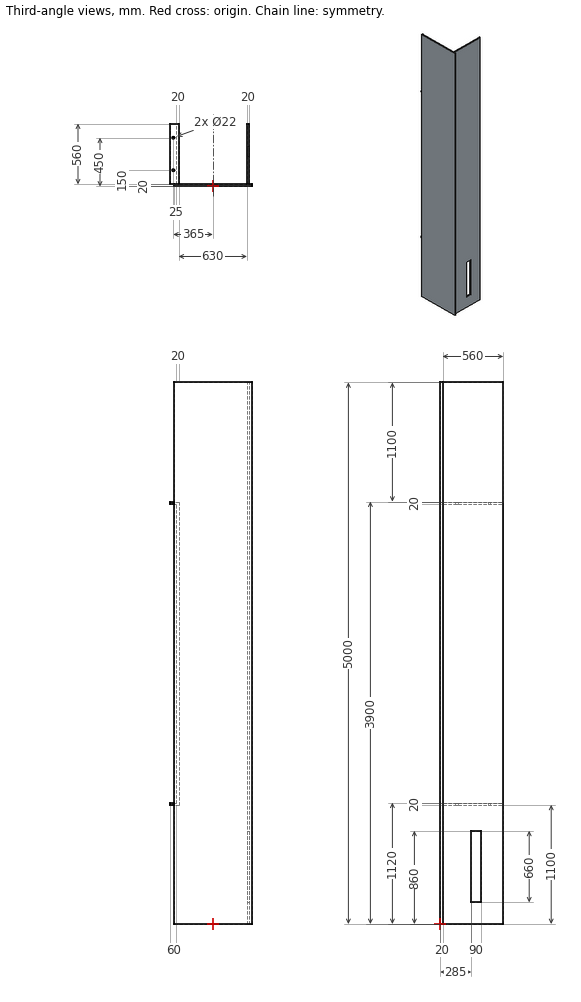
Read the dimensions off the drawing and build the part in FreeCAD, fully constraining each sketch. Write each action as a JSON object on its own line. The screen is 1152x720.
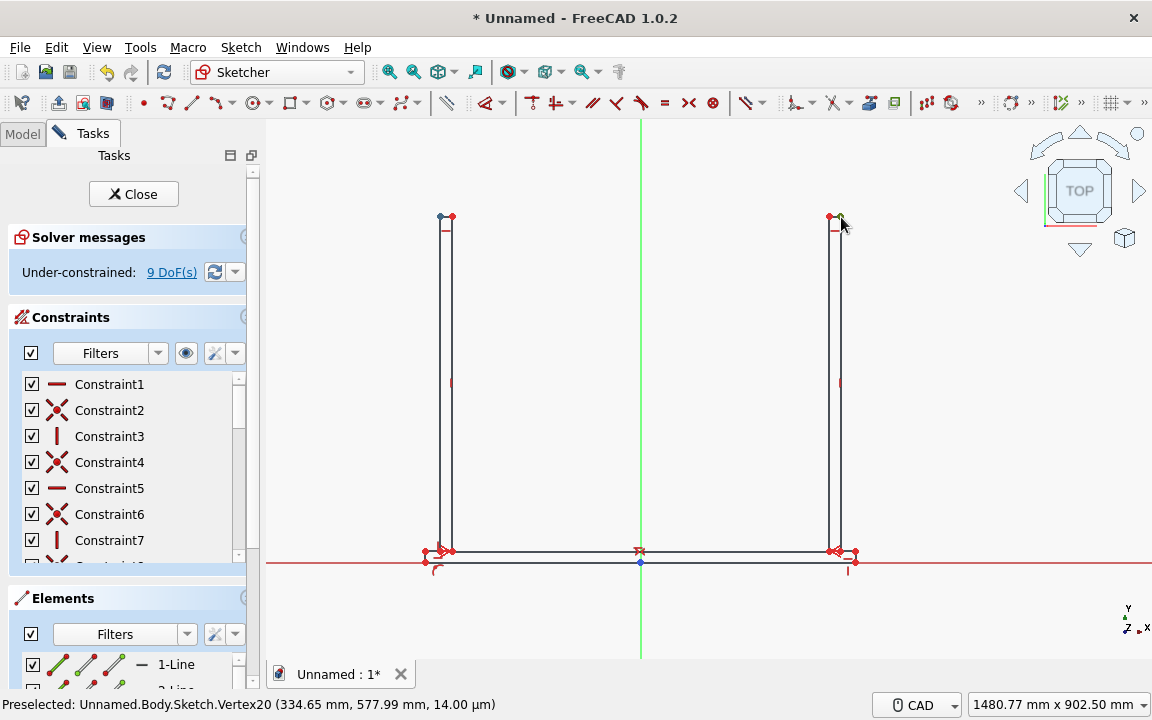
{"action": "left_click", "coordinate": [641, 596]}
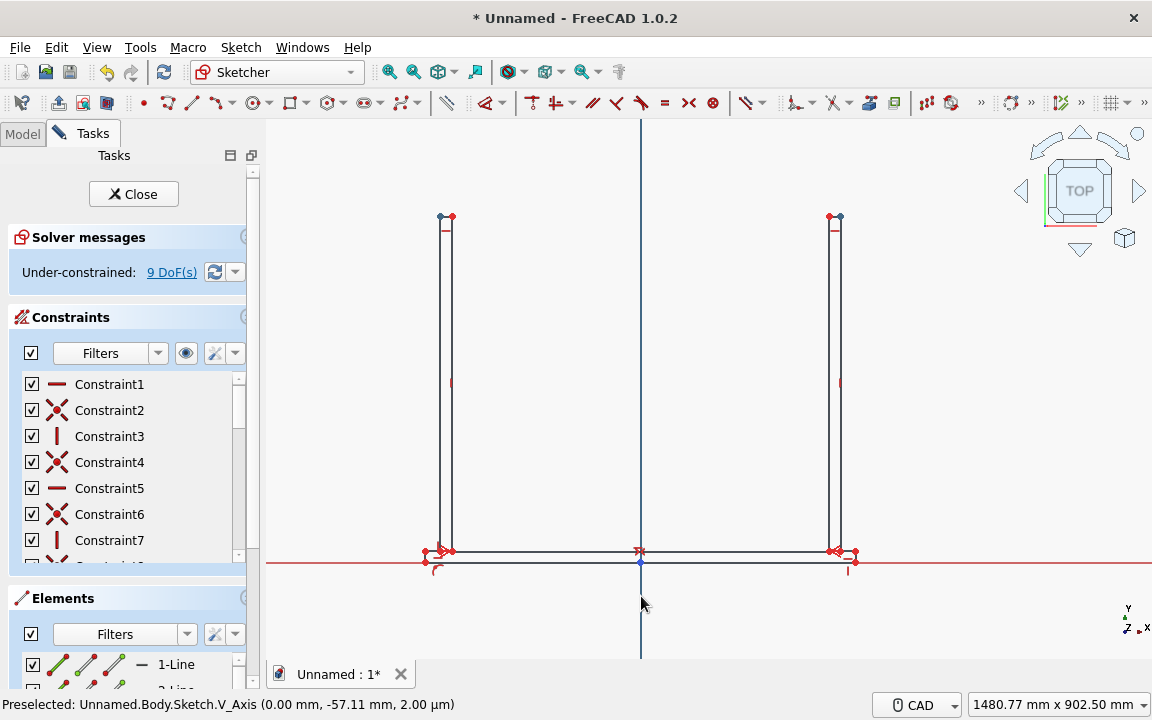
{"action": "left_click", "coordinate": [690, 104]}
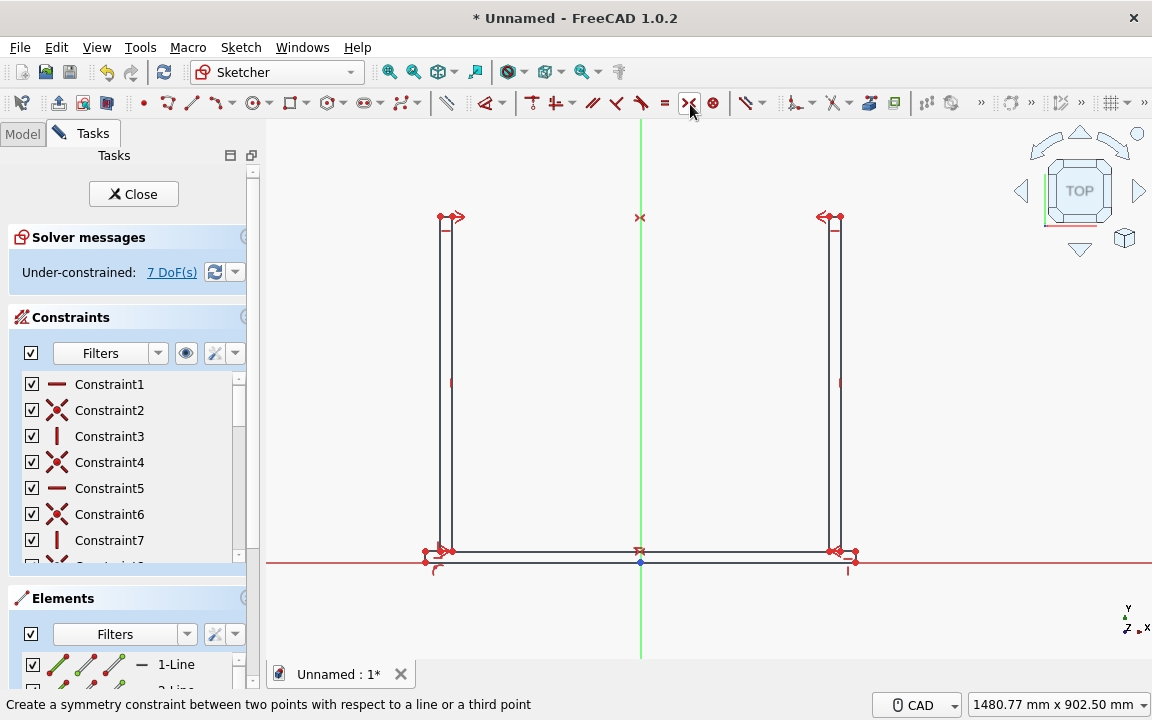
{"action": "scroll", "coordinate": [446, 217], "scroll_direction": "up", "scroll_amount": 6}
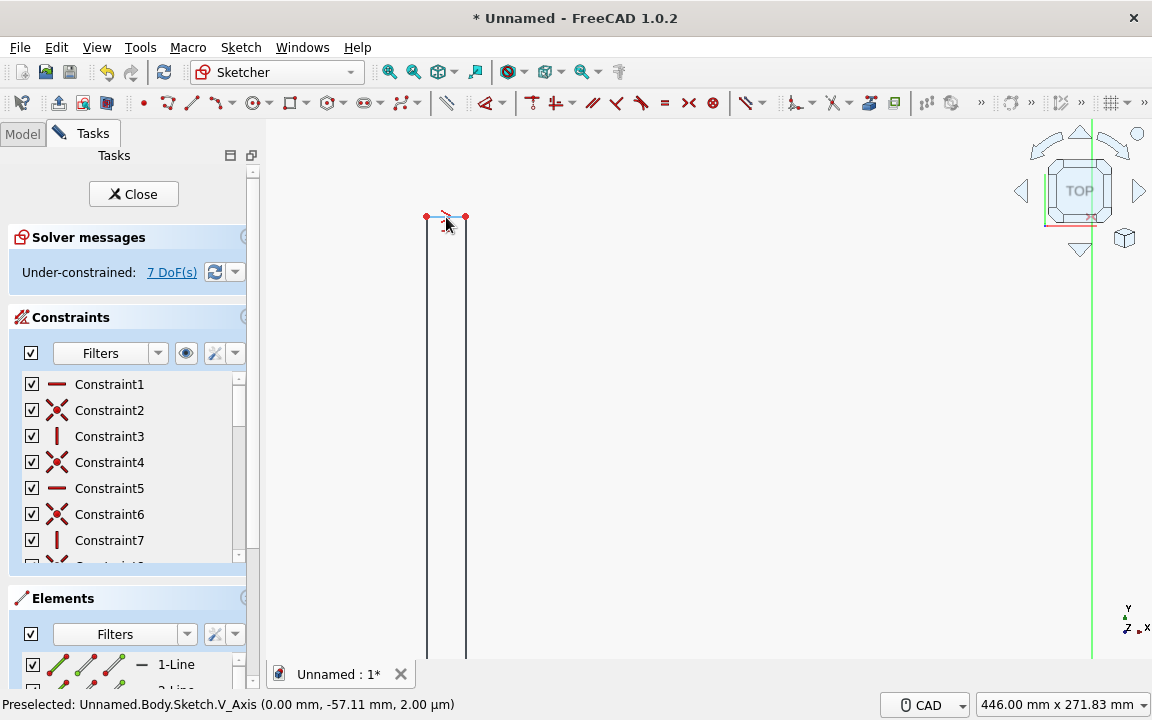
{"action": "left_click", "coordinate": [446, 217]}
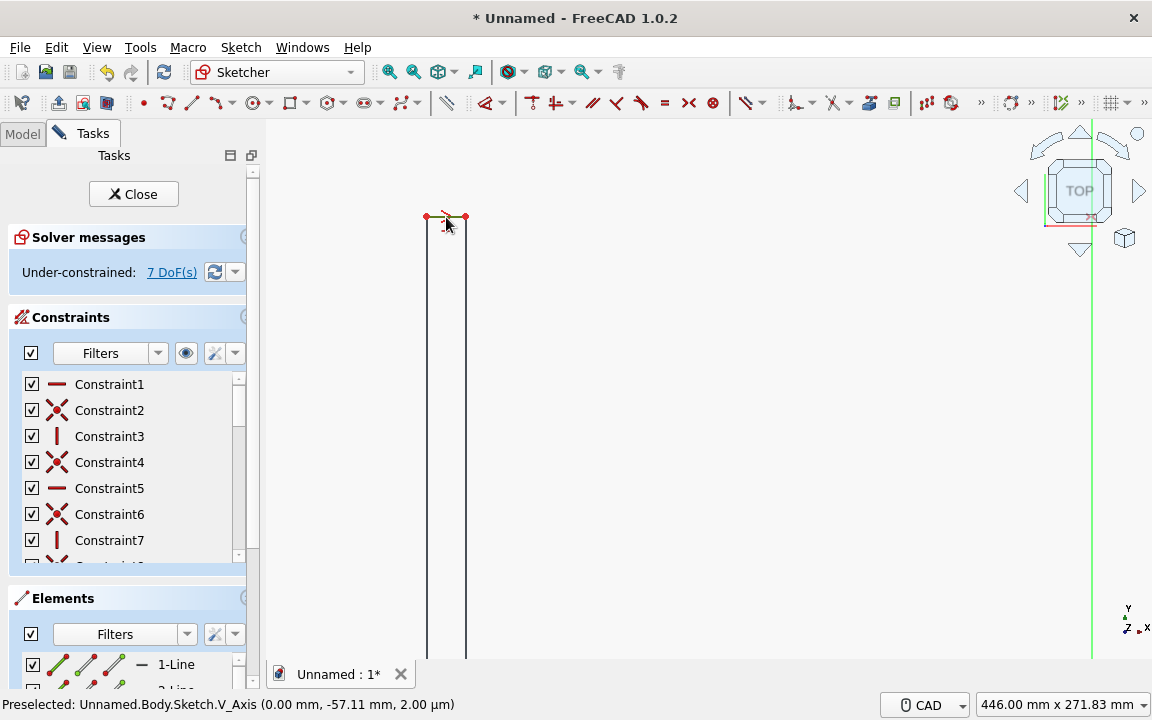
{"action": "key", "text": "l"}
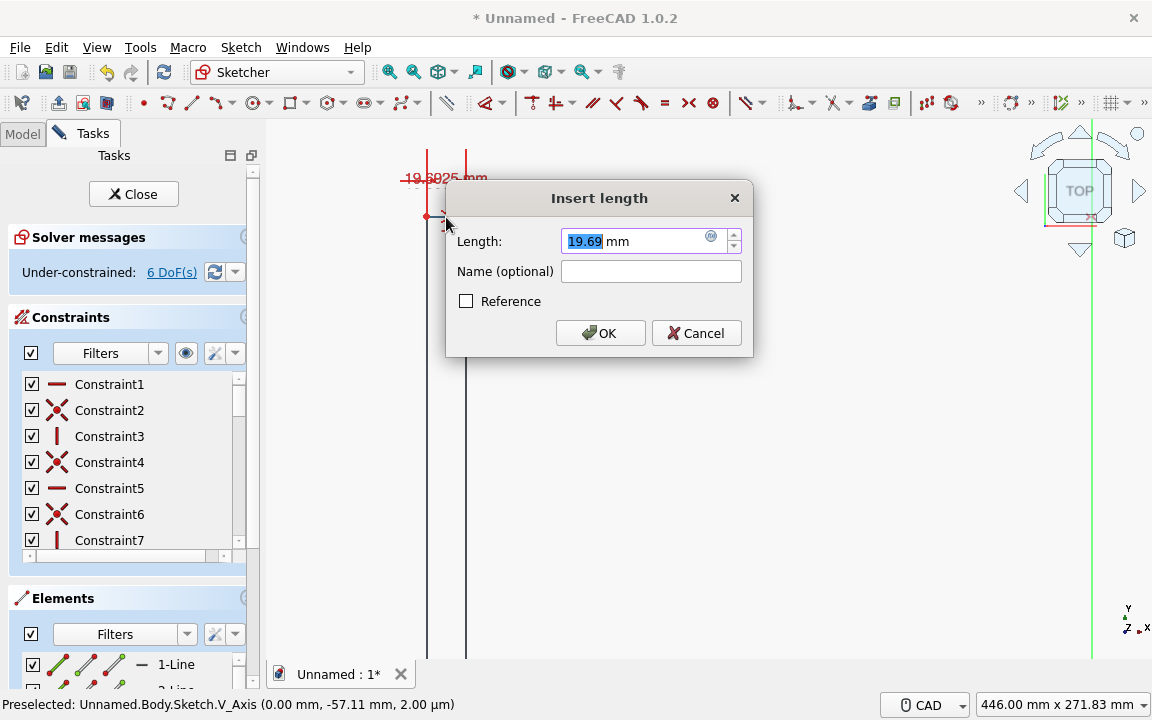
{"action": "type", "text": "20"}
{"action": "key", "text": "Return"}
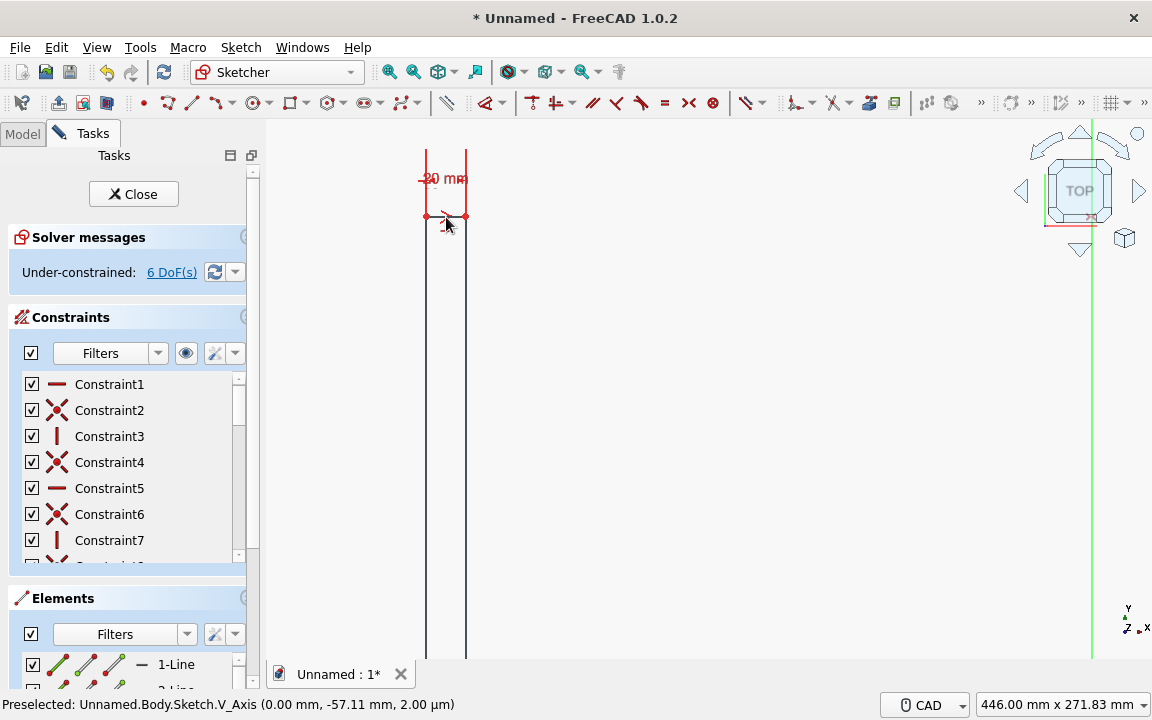
{"action": "scroll", "coordinate": [446, 217], "scroll_direction": "down", "scroll_amount": 6}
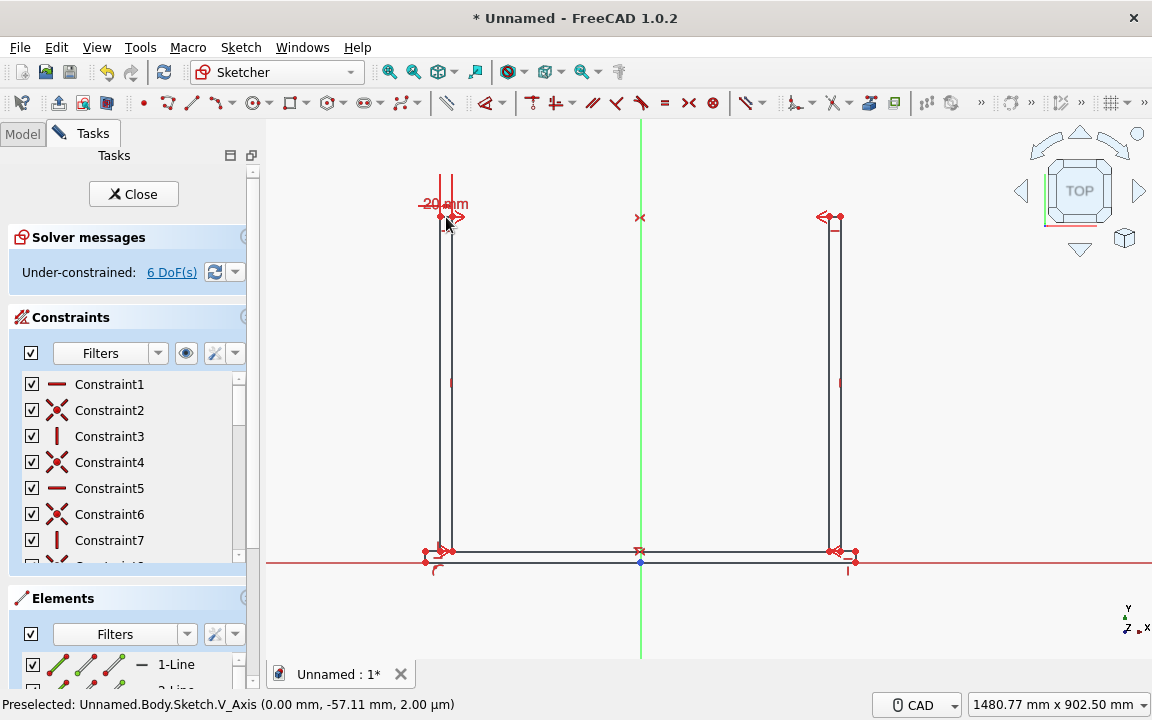
{"action": "scroll", "coordinate": [436, 551], "scroll_direction": "up", "scroll_amount": 6}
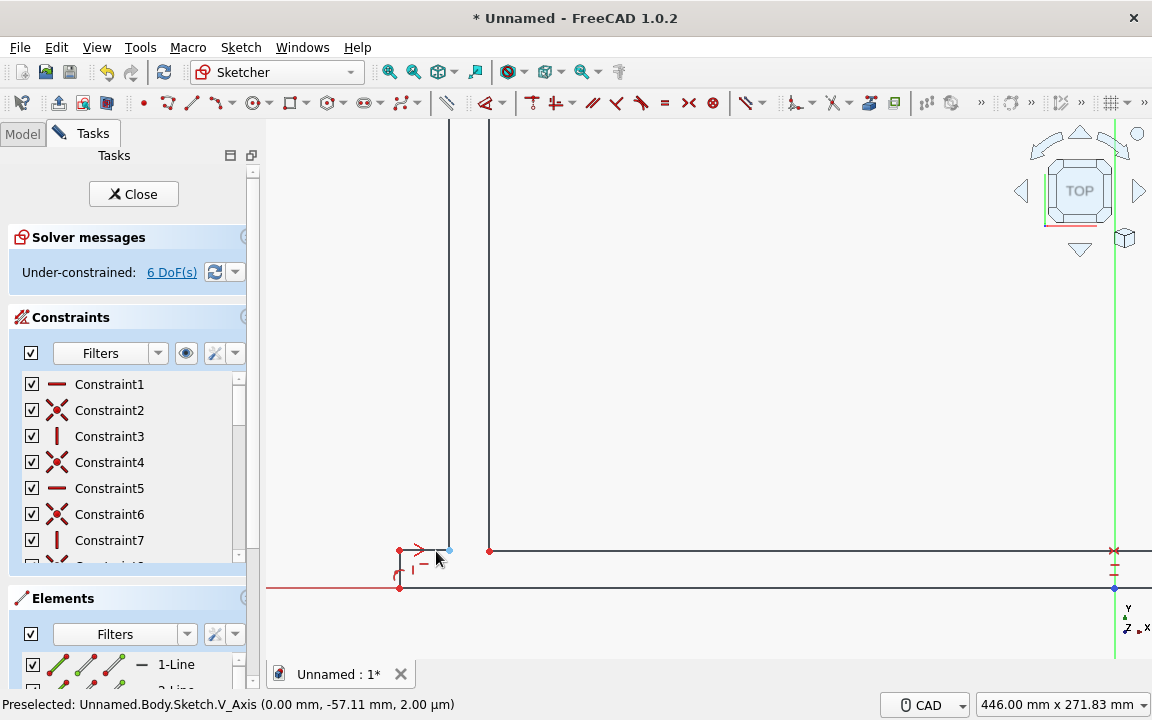
{"action": "left_click", "coordinate": [434, 550]}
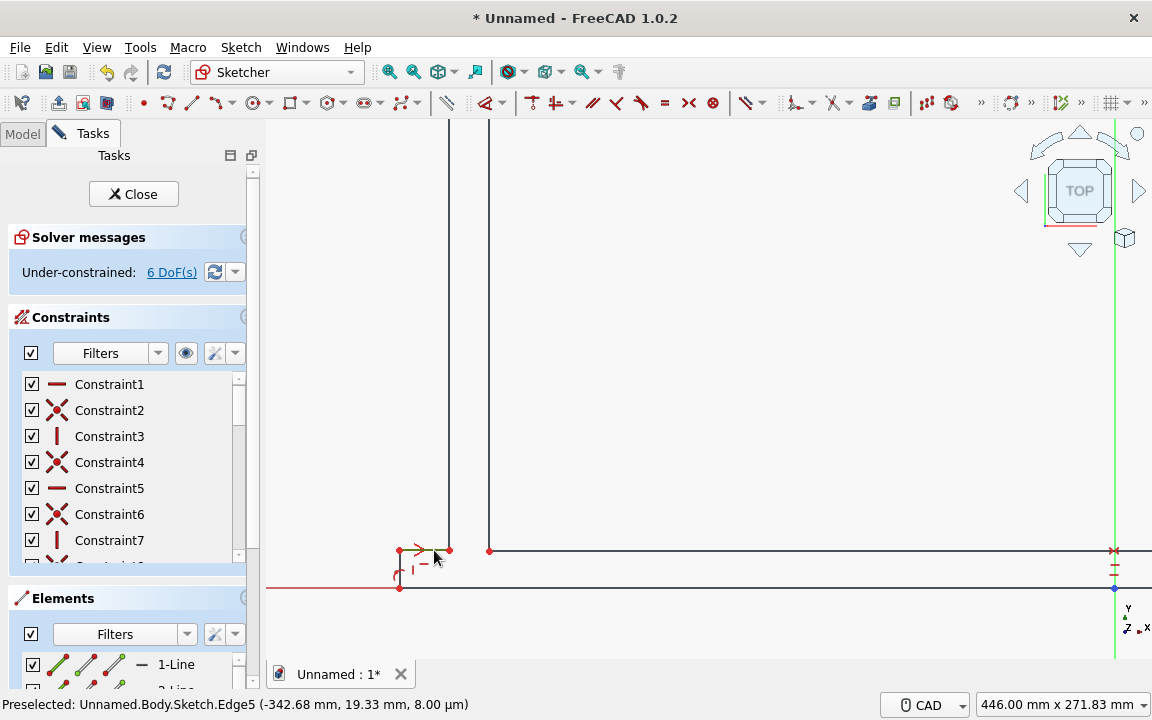
{"action": "left_click", "coordinate": [504, 104]}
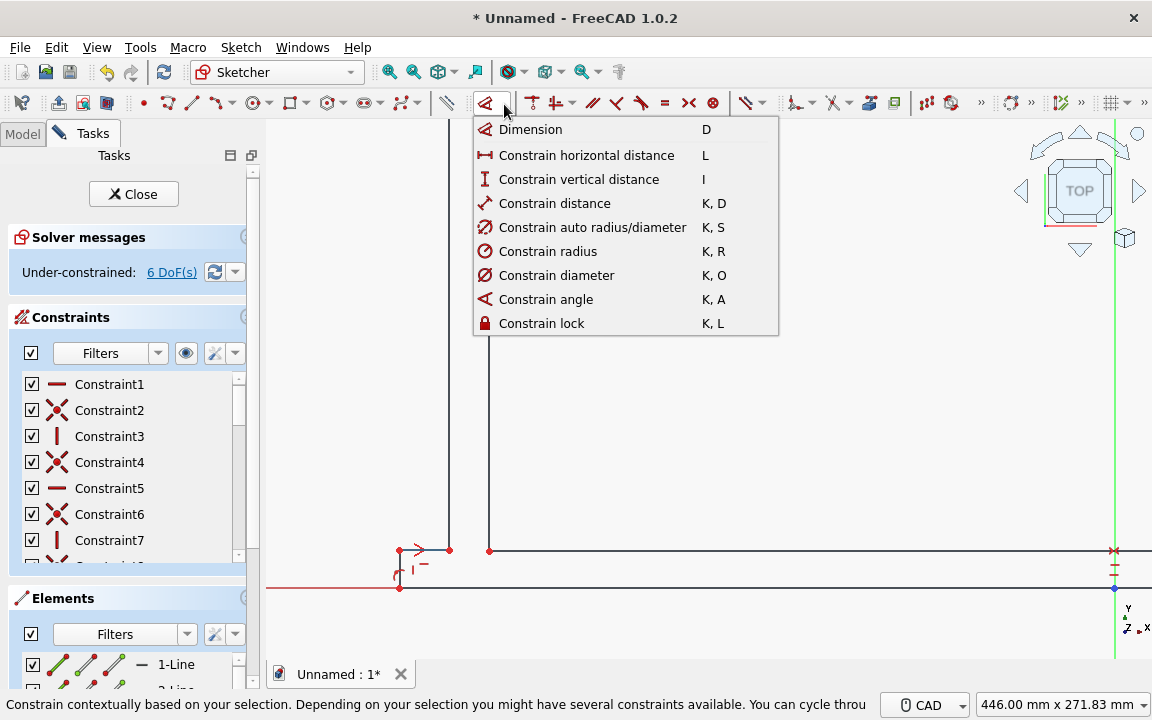
{"action": "left_click", "coordinate": [626, 155]}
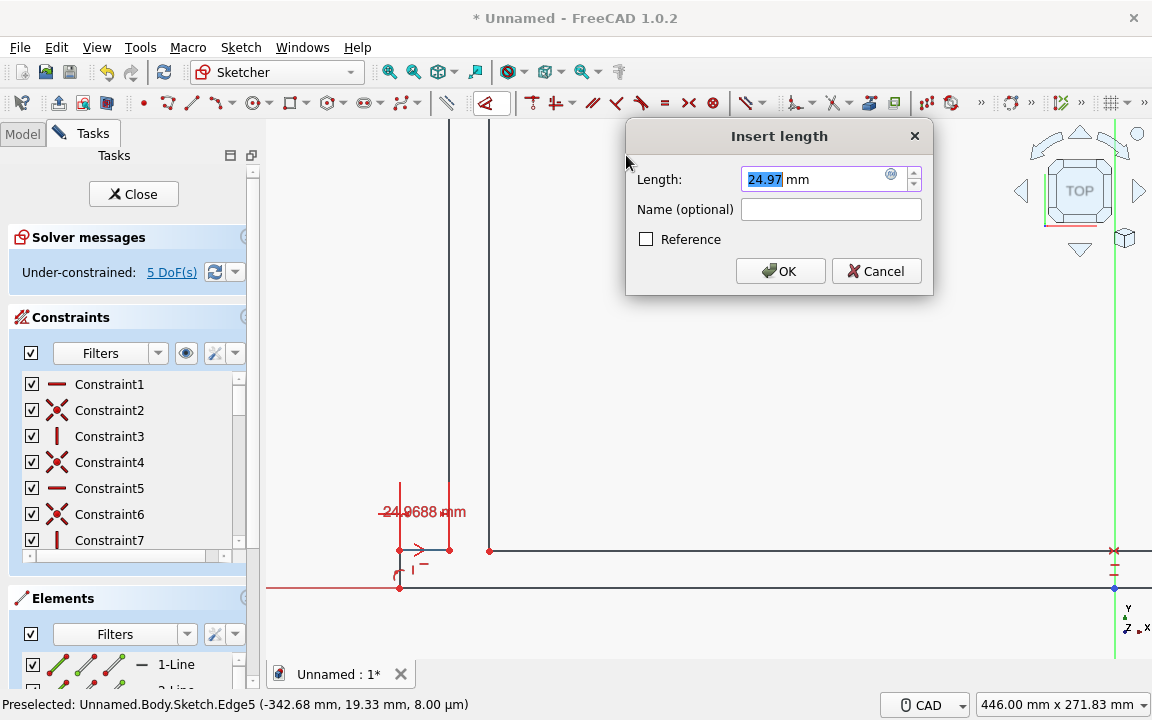
{"action": "type", "text": "25"}
{"action": "key", "text": "Return"}